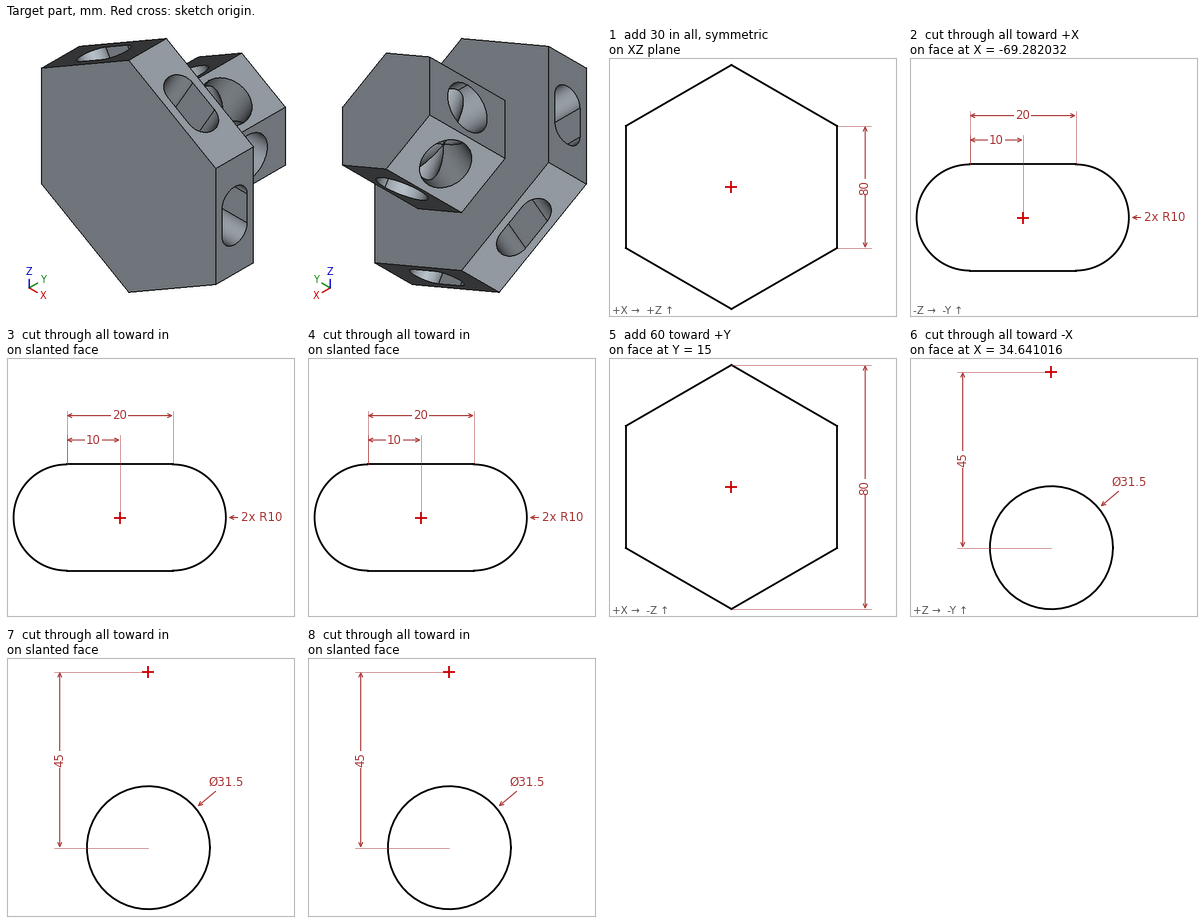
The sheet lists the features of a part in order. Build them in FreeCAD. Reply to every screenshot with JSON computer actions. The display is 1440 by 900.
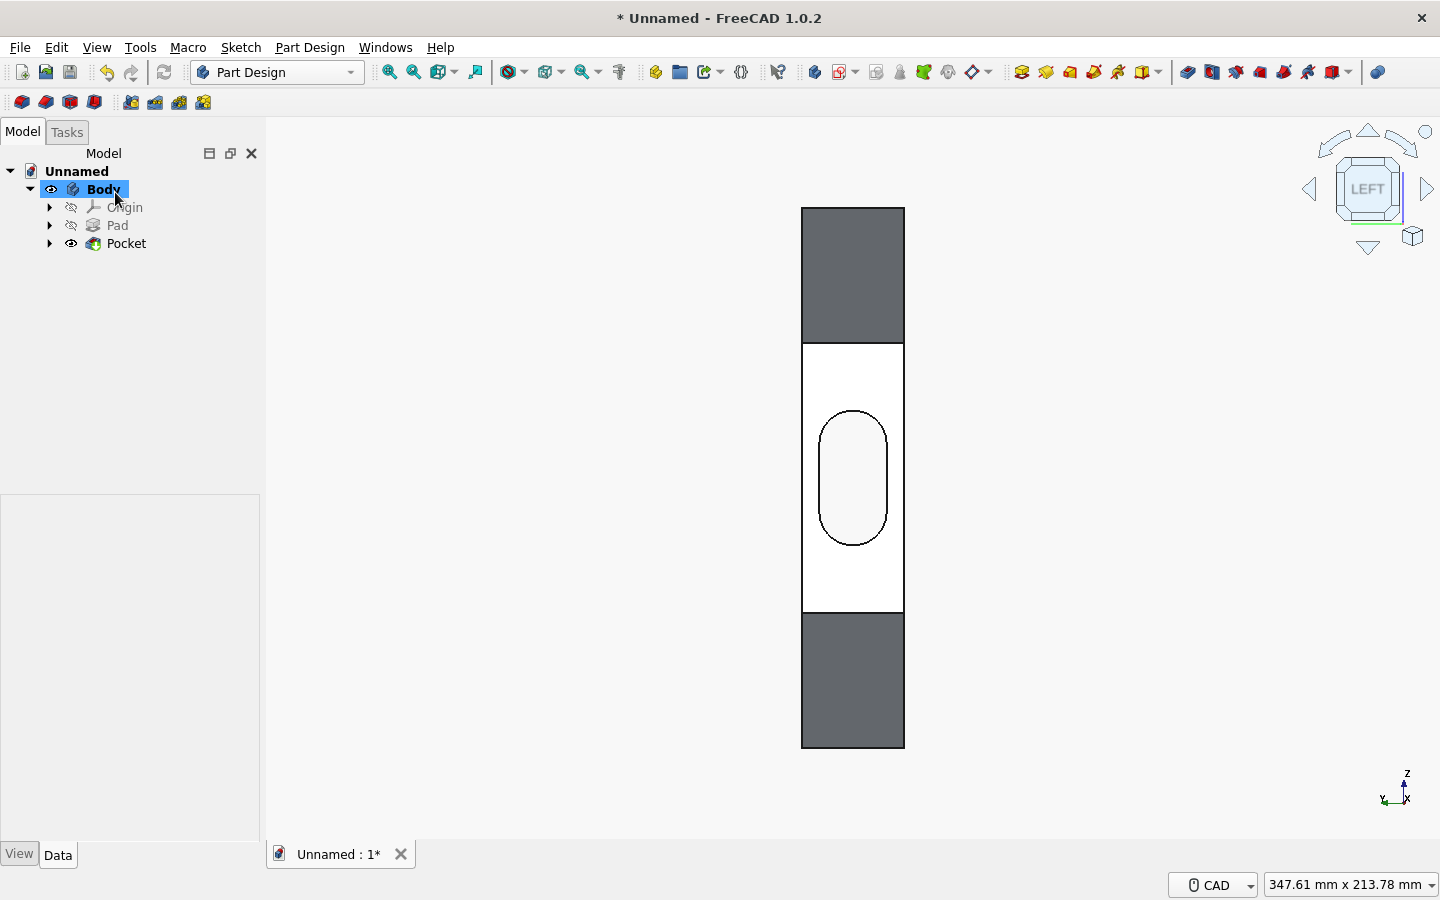
{"action": "key", "text": "5"}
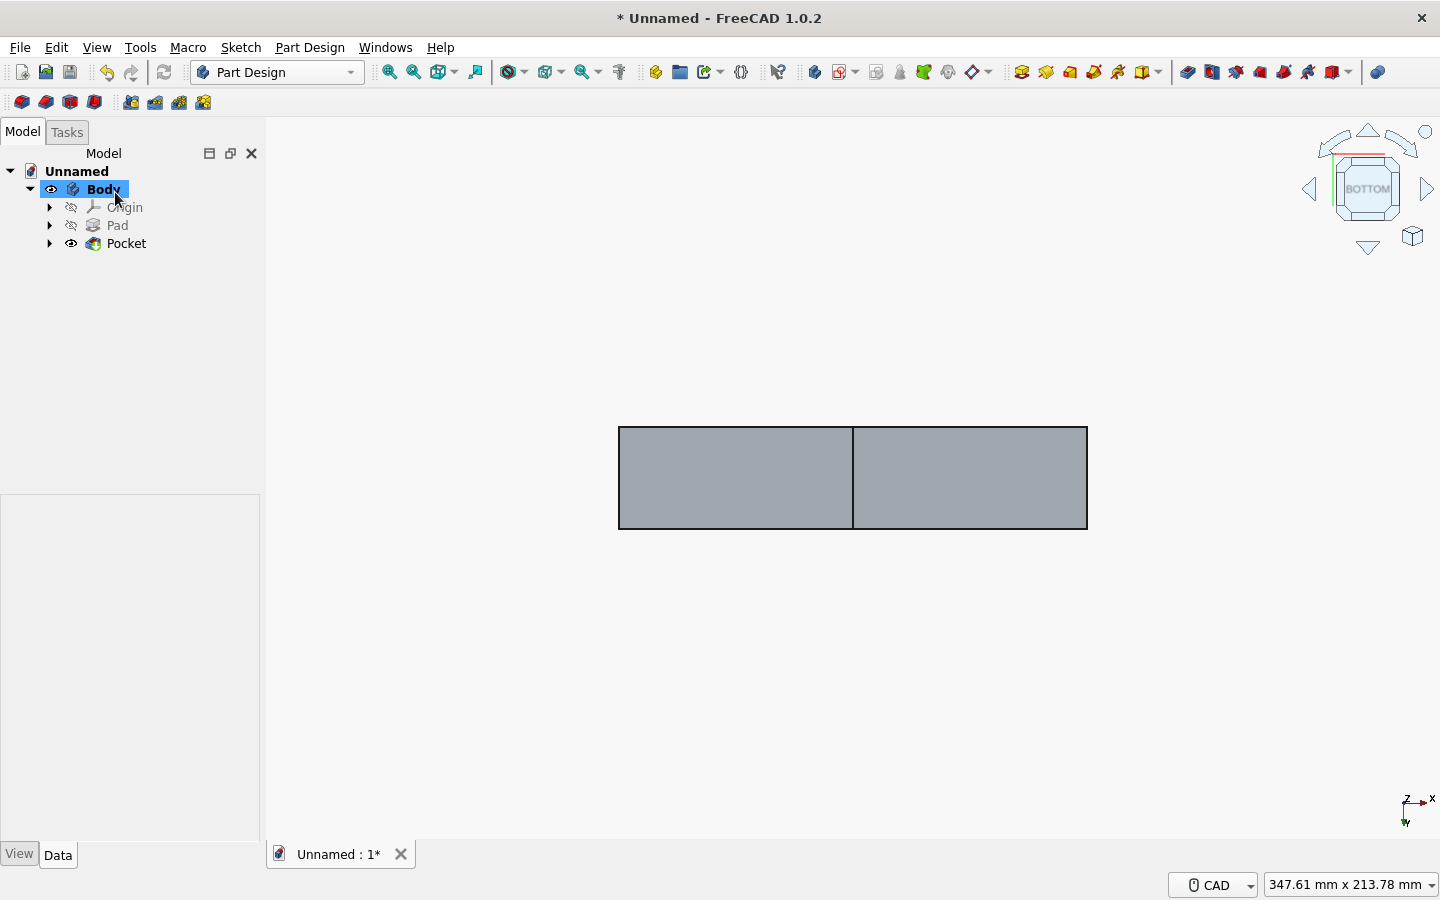
{"action": "left_click", "coordinate": [390, 72]}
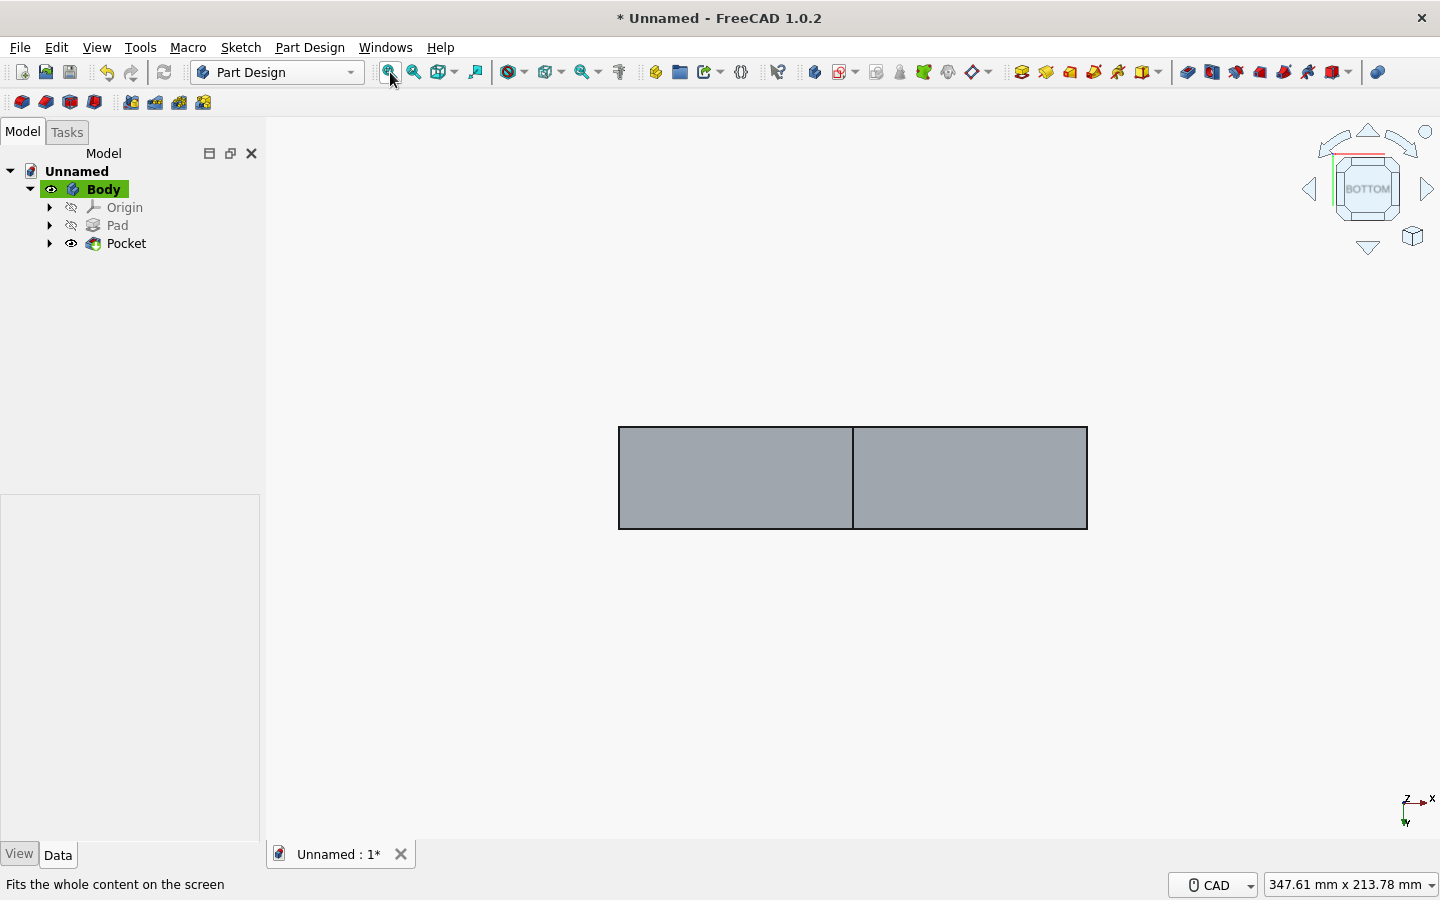
{"action": "left_click", "coordinate": [1037, 477]}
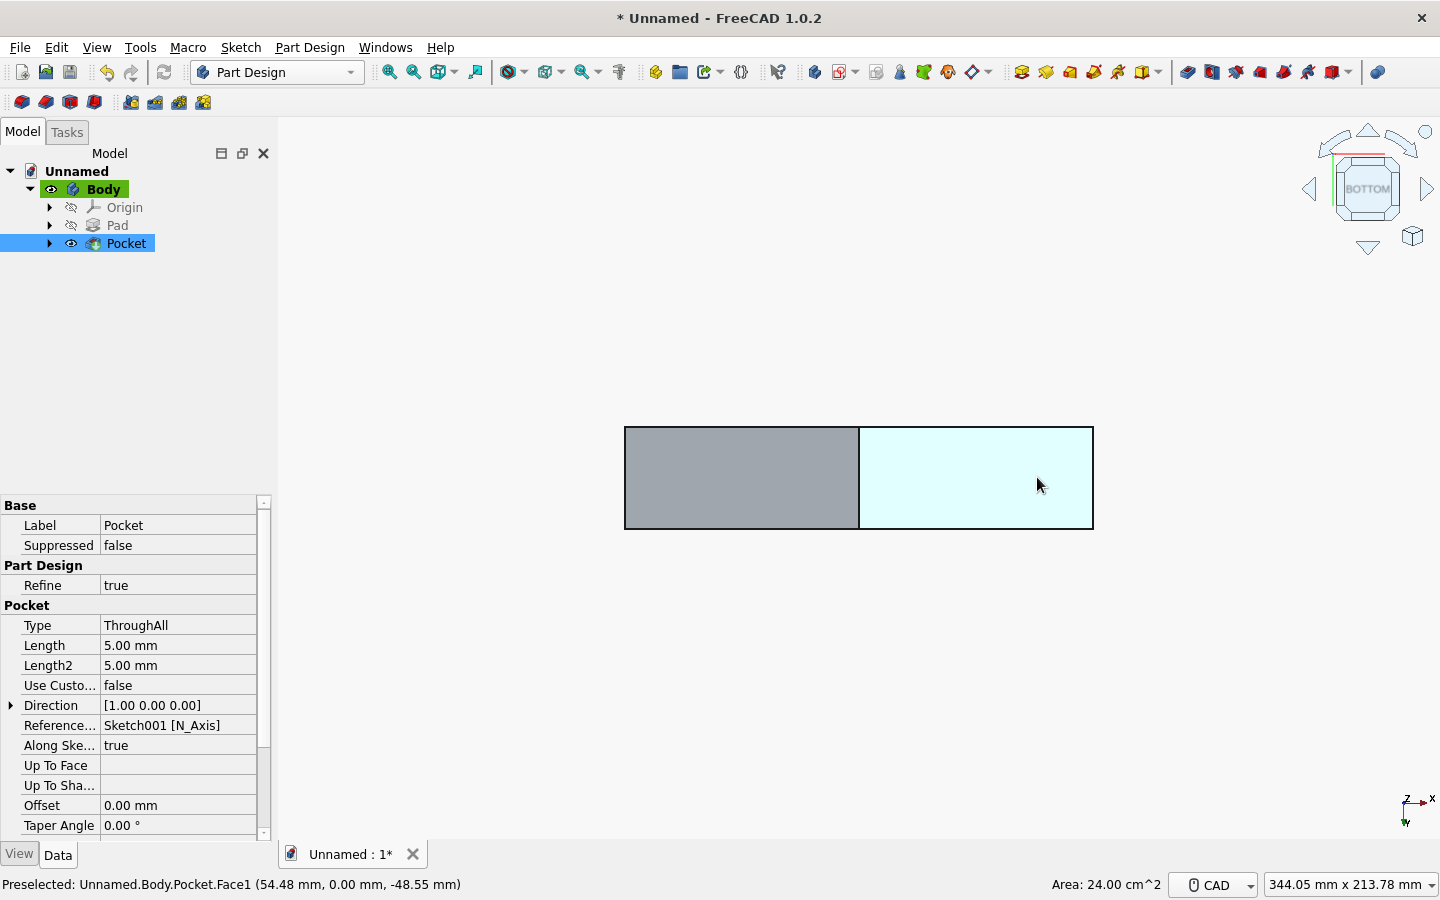
{"action": "left_click", "coordinate": [840, 72]}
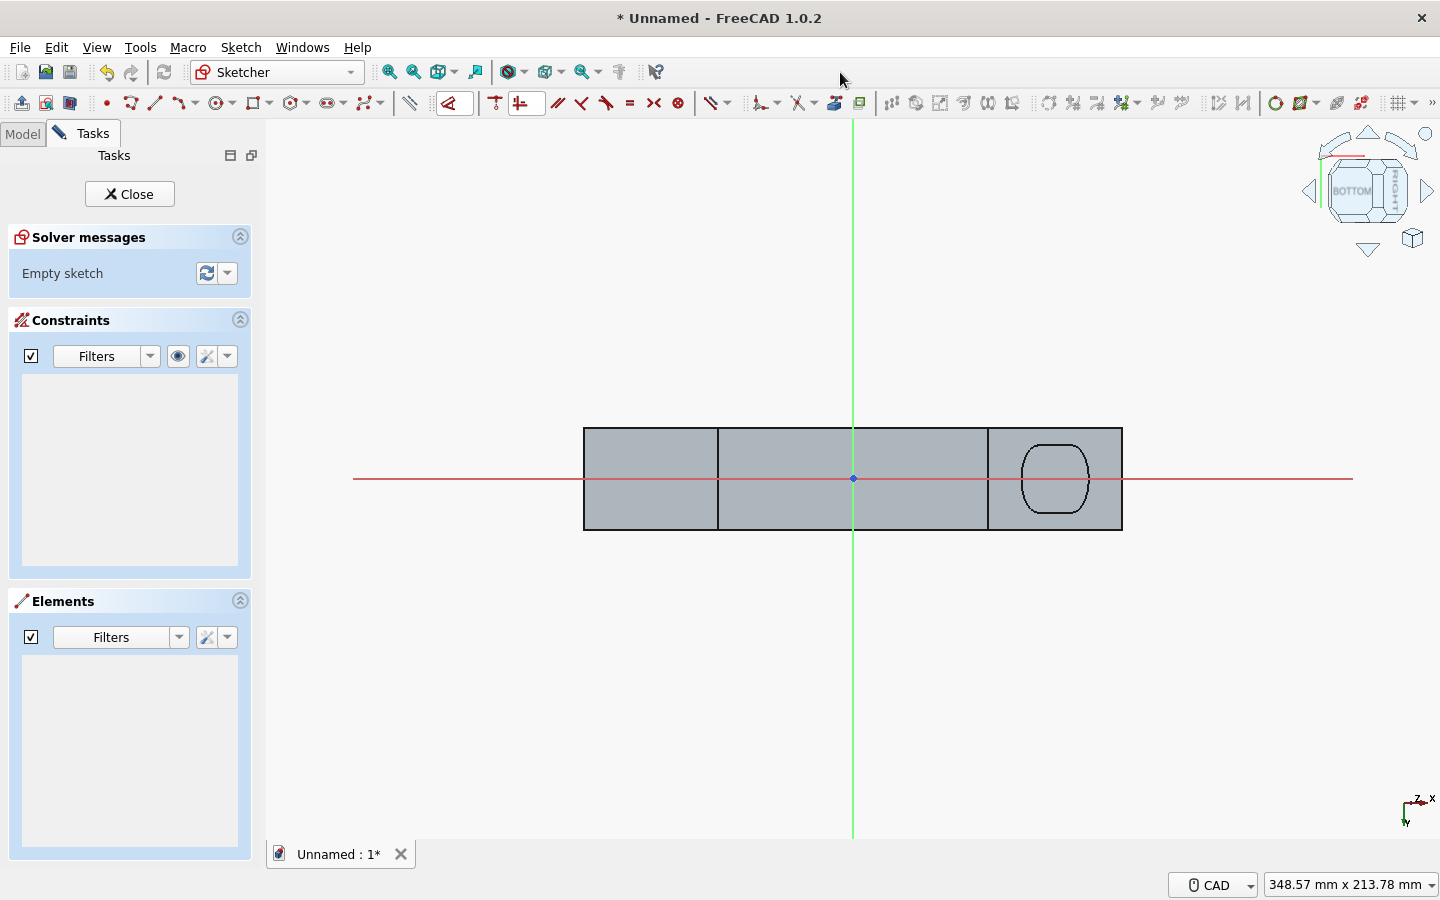
{"action": "scroll", "coordinate": [870, 479], "scroll_direction": "up", "scroll_amount": 8}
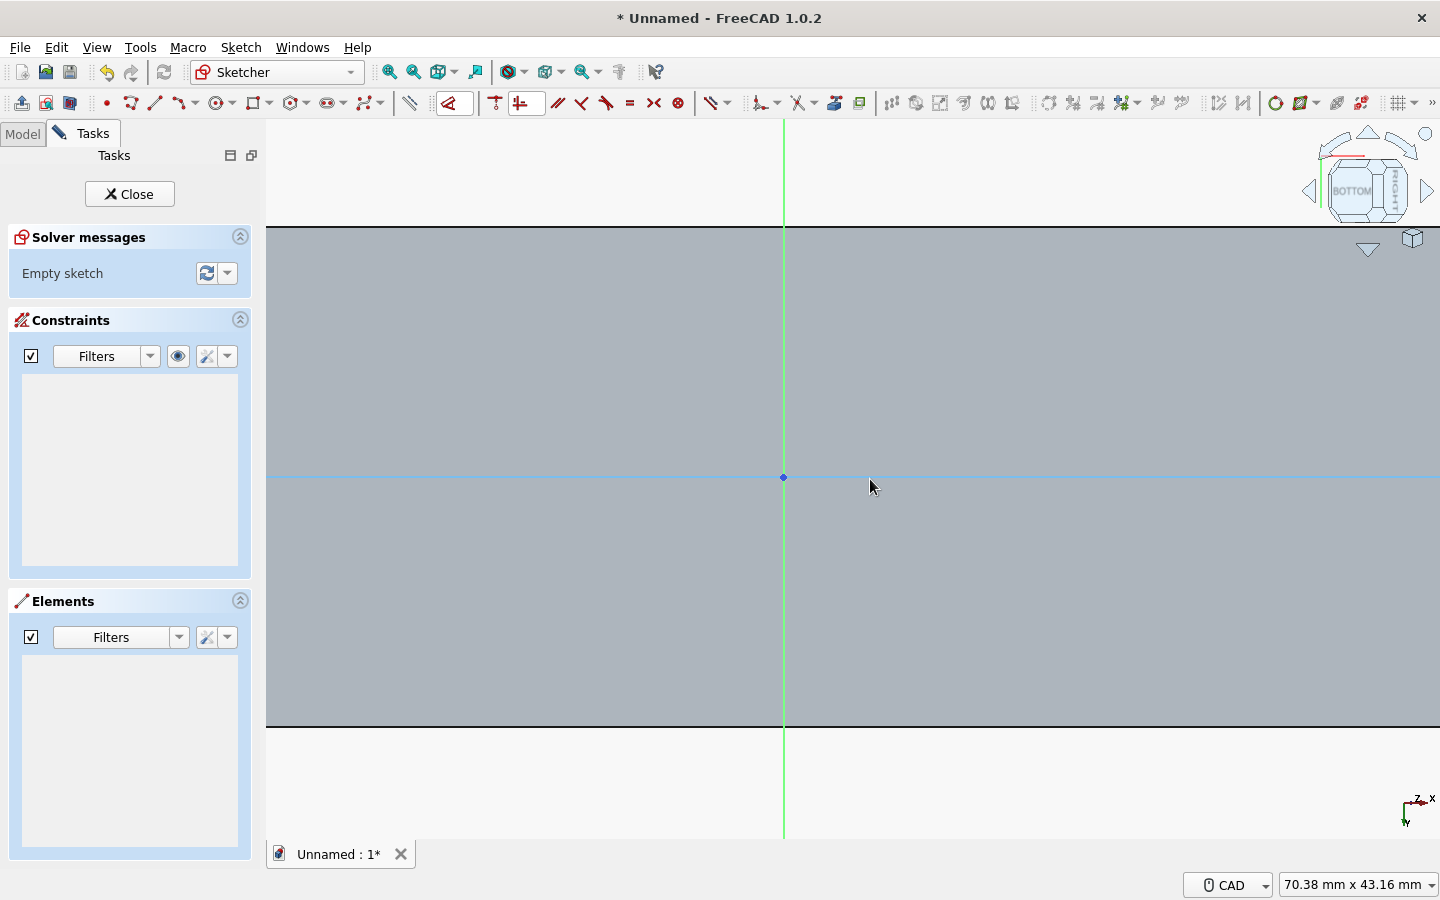
{"action": "left_click", "coordinate": [328, 104]}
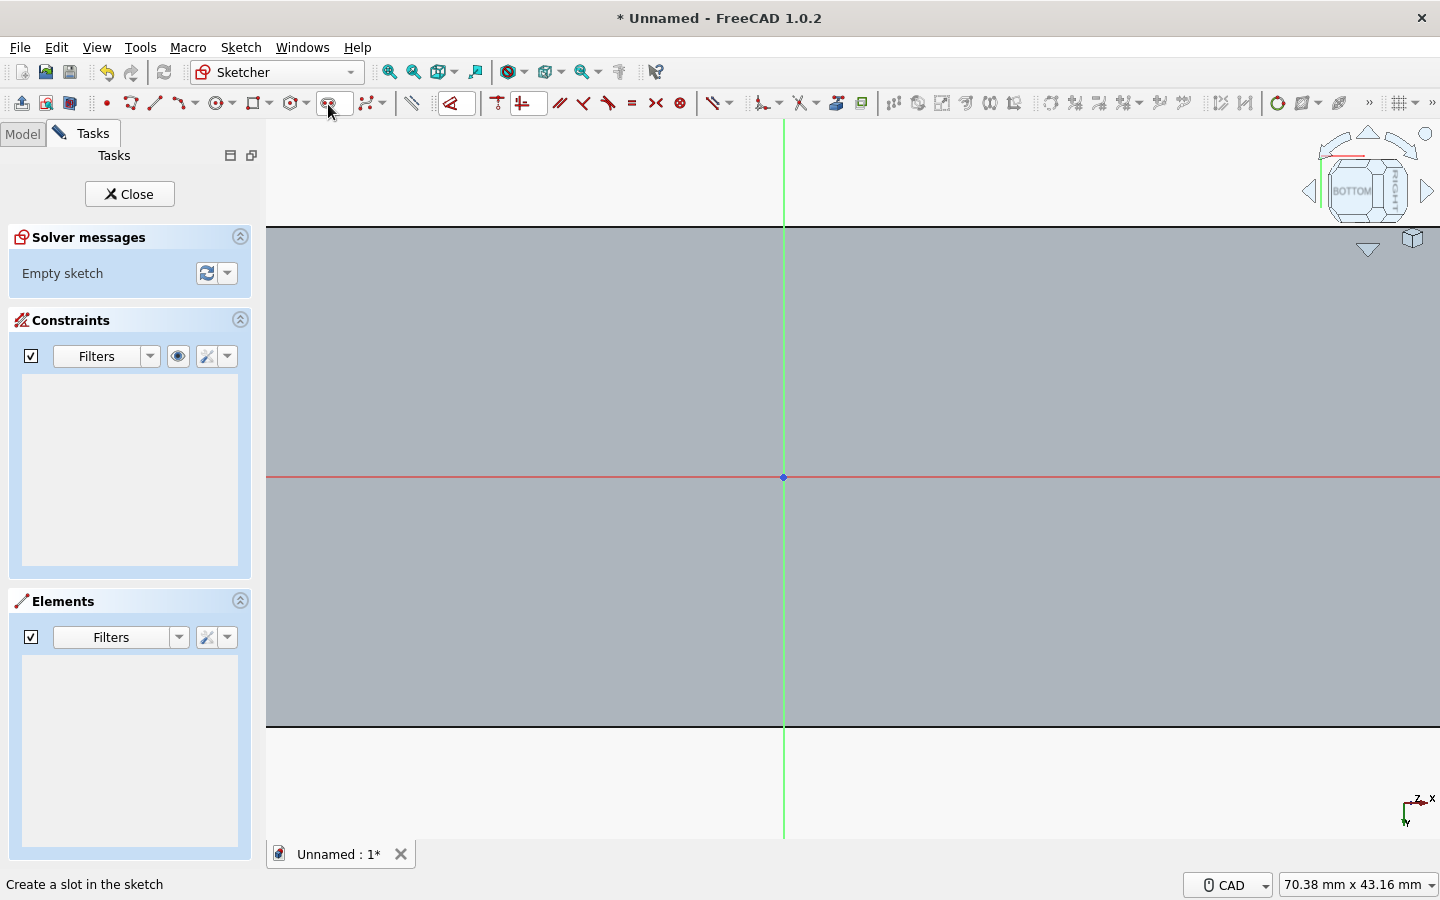
{"action": "left_click", "coordinate": [617, 477]}